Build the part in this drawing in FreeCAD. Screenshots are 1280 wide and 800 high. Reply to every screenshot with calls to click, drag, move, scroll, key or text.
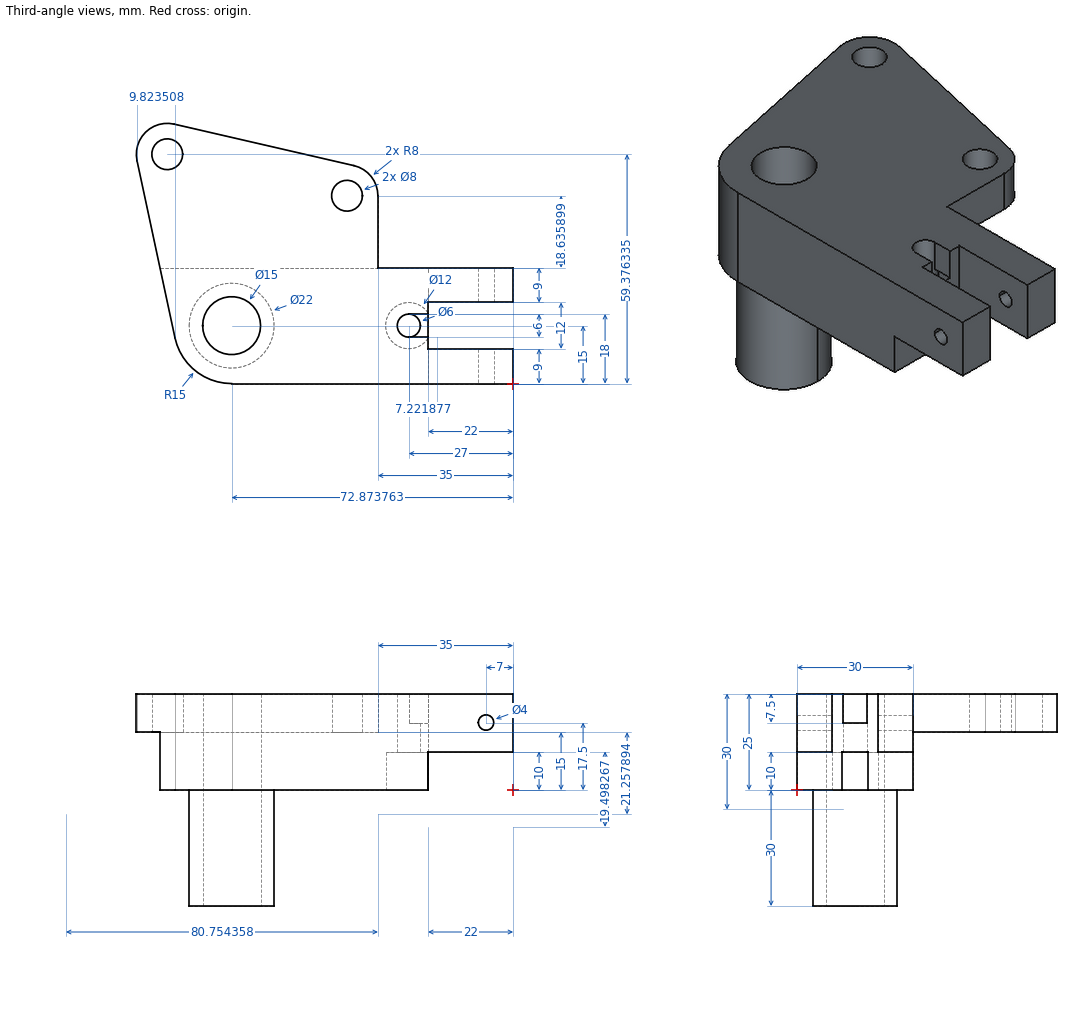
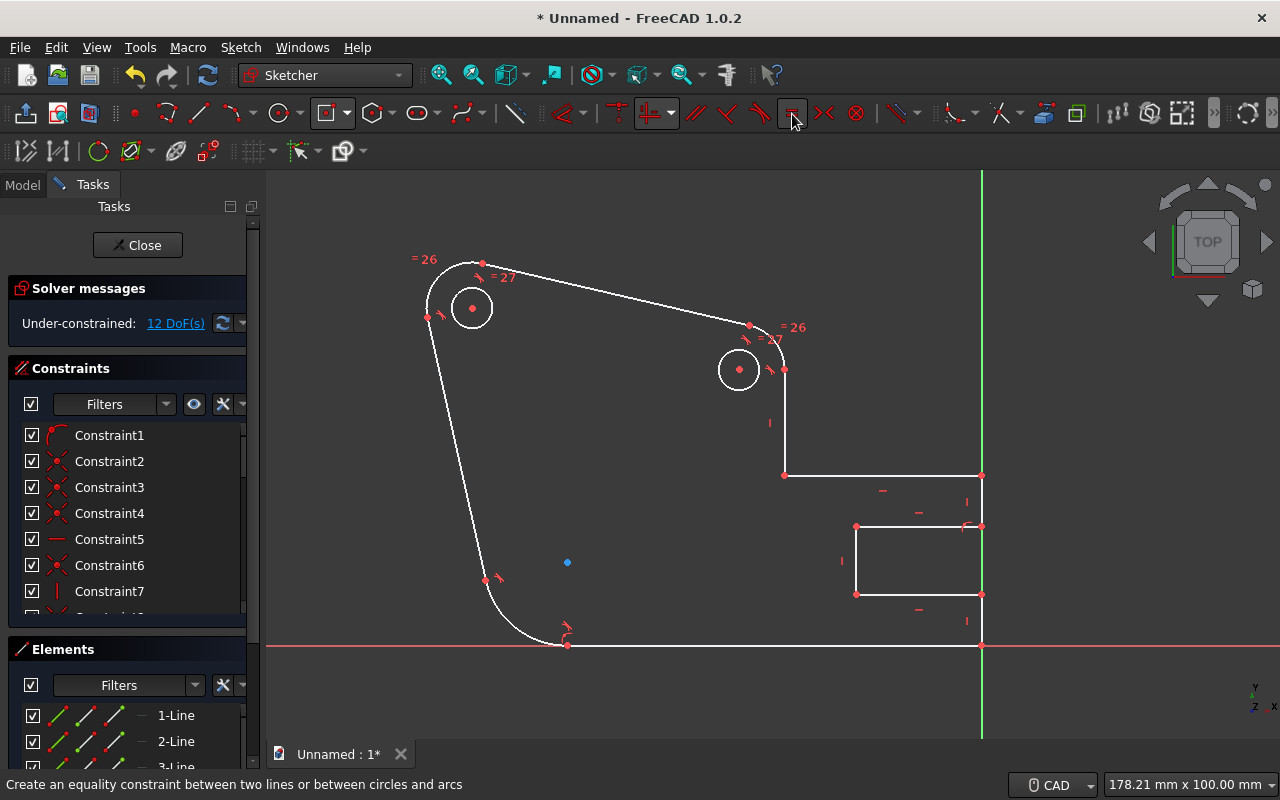
click(562, 114)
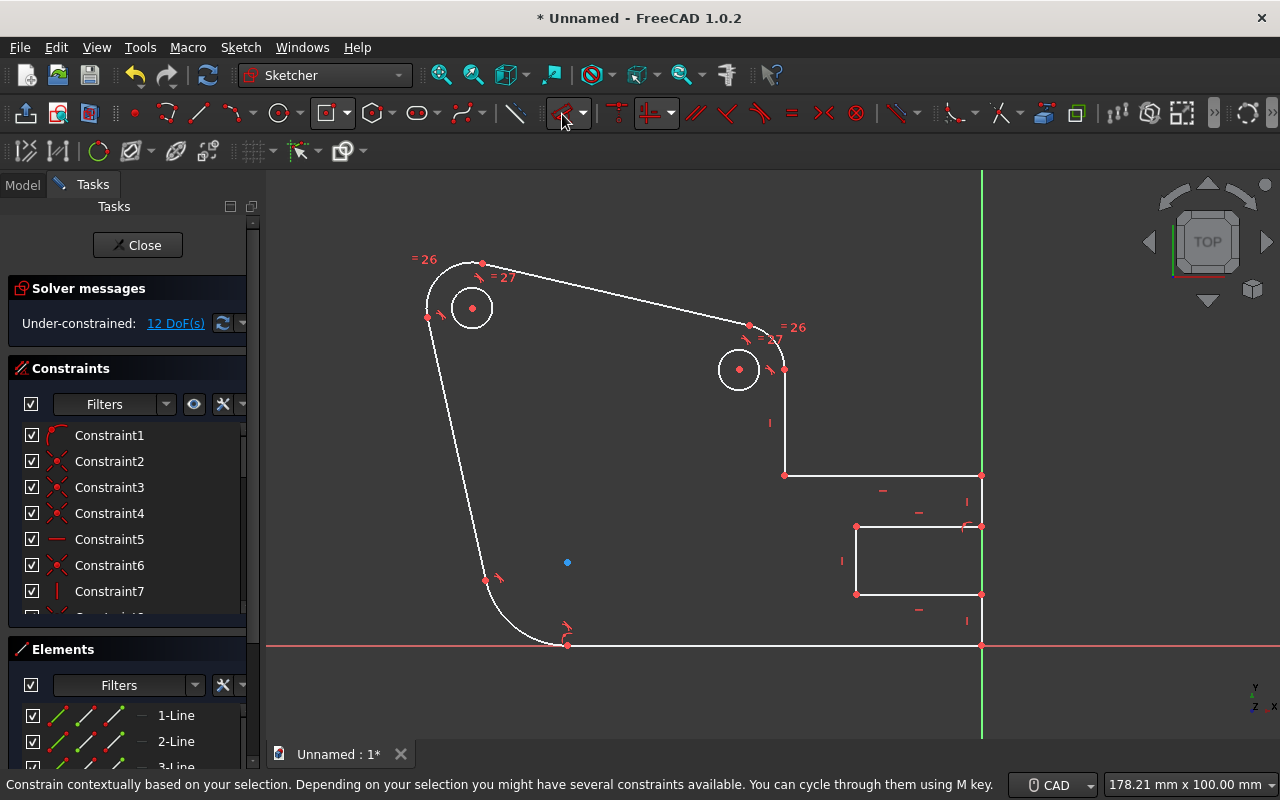
click(781, 352)
click(810, 339)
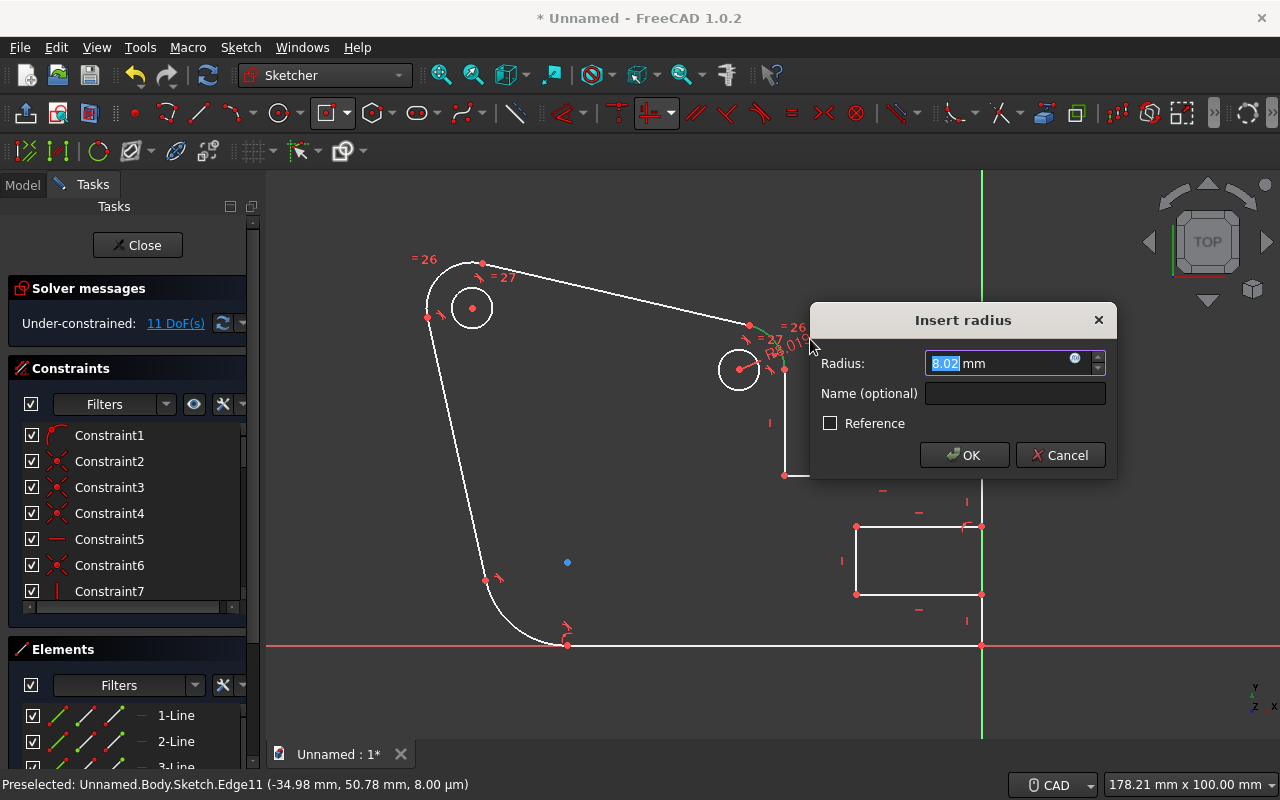
text(8)
key(Return)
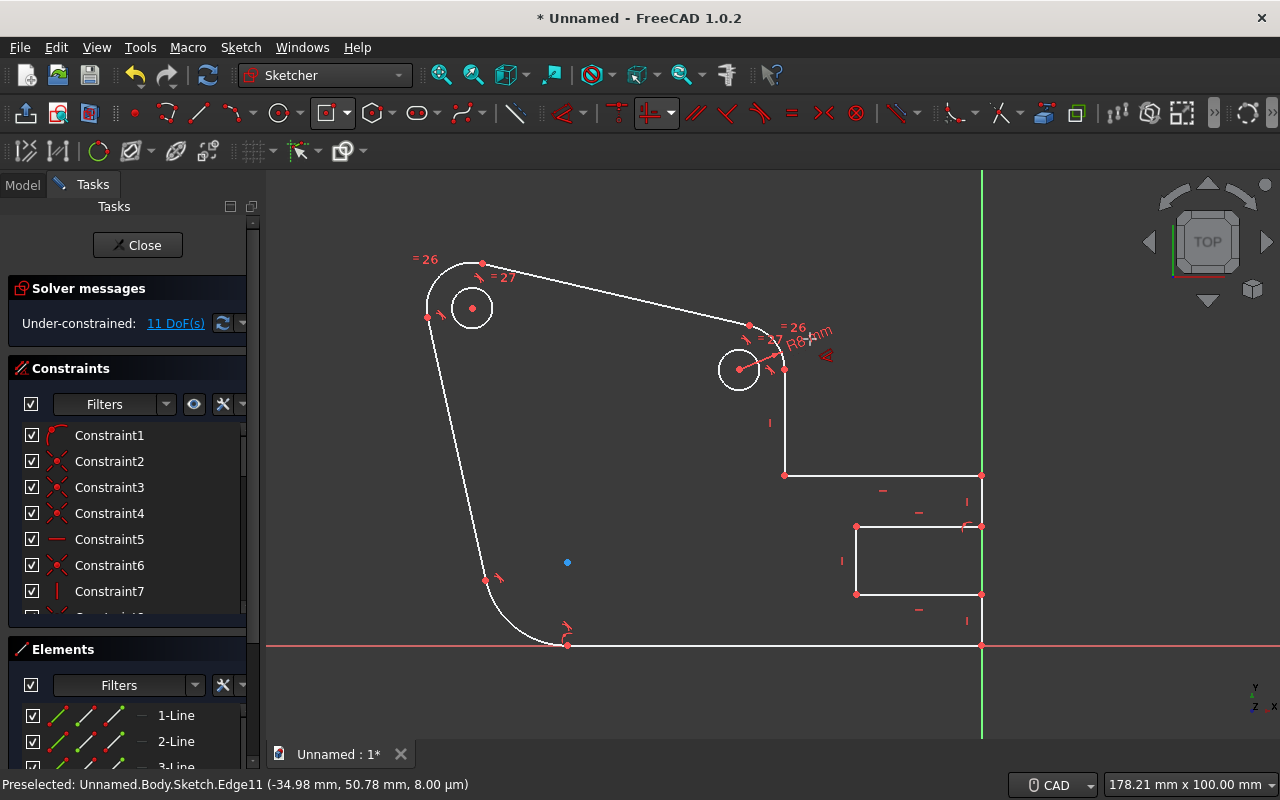
click(500, 611)
click(474, 630)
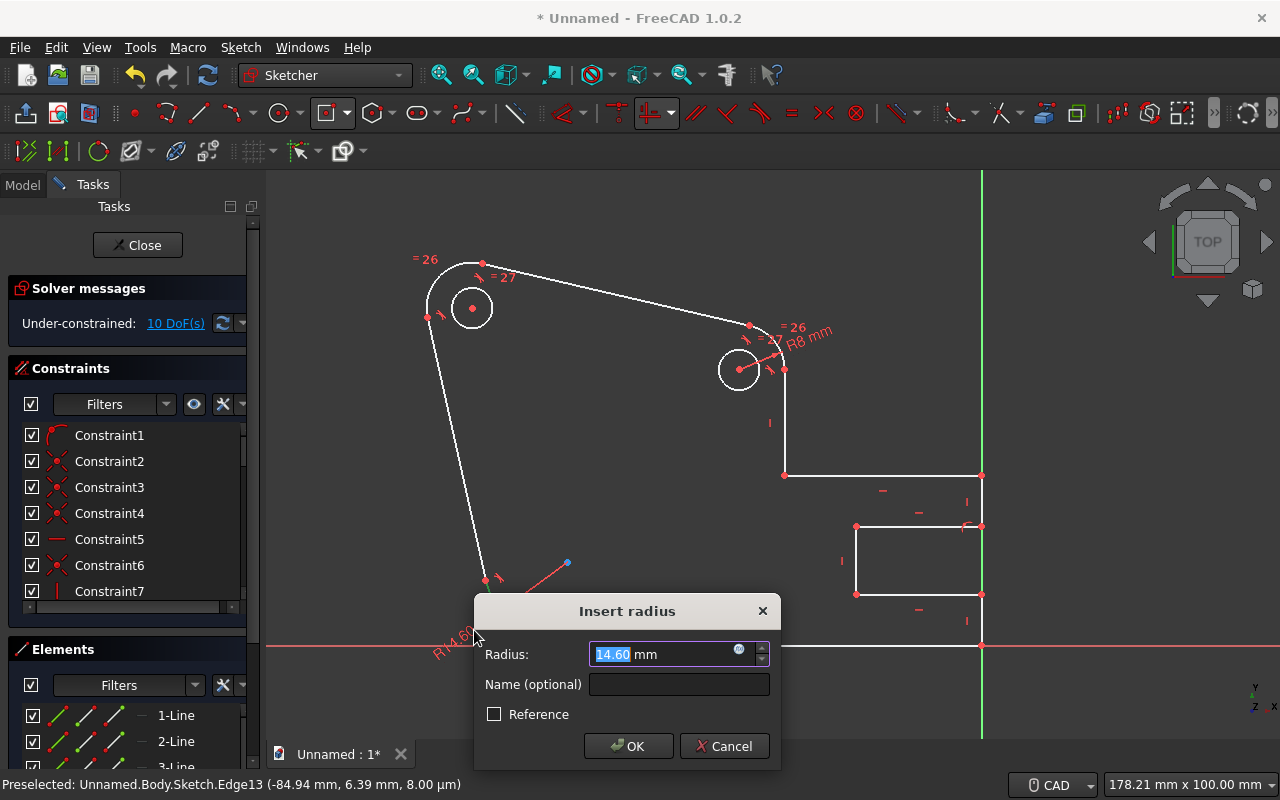
text(15)
key(Return)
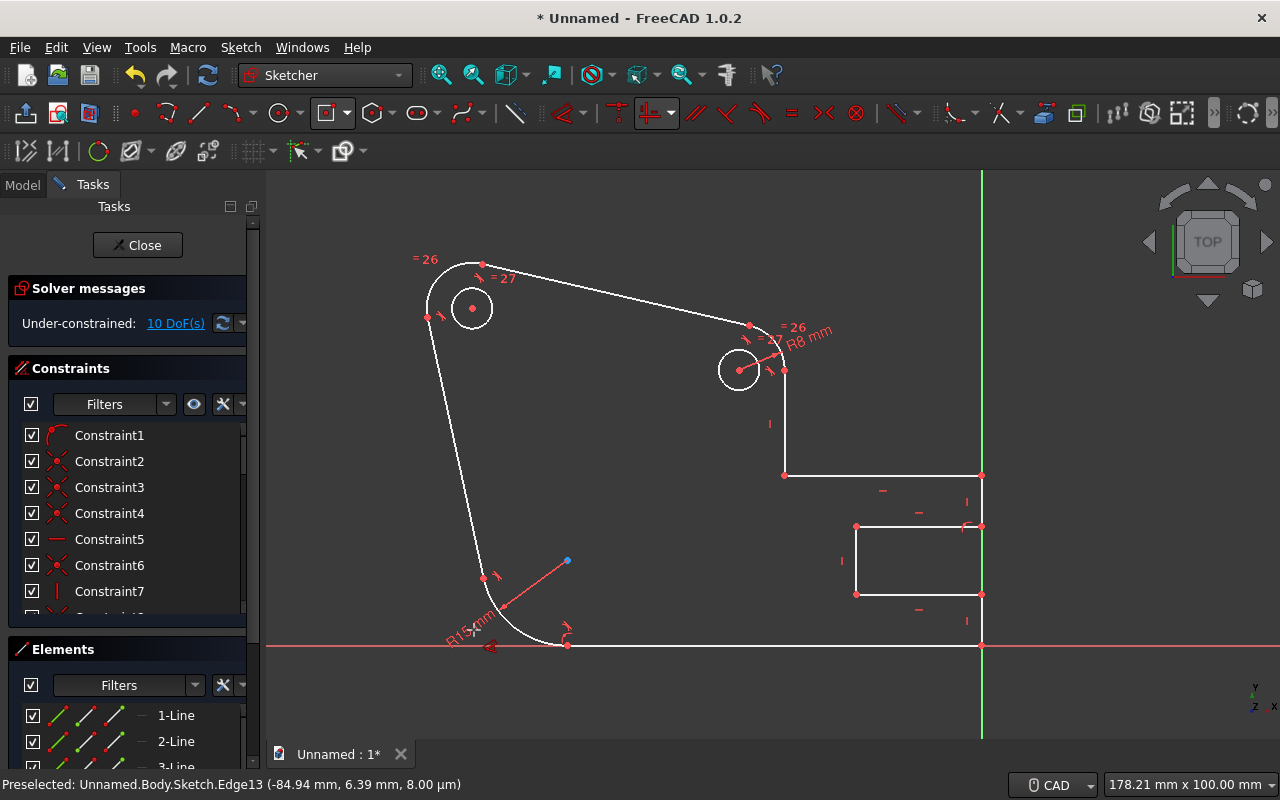
click(753, 356)
click(702, 334)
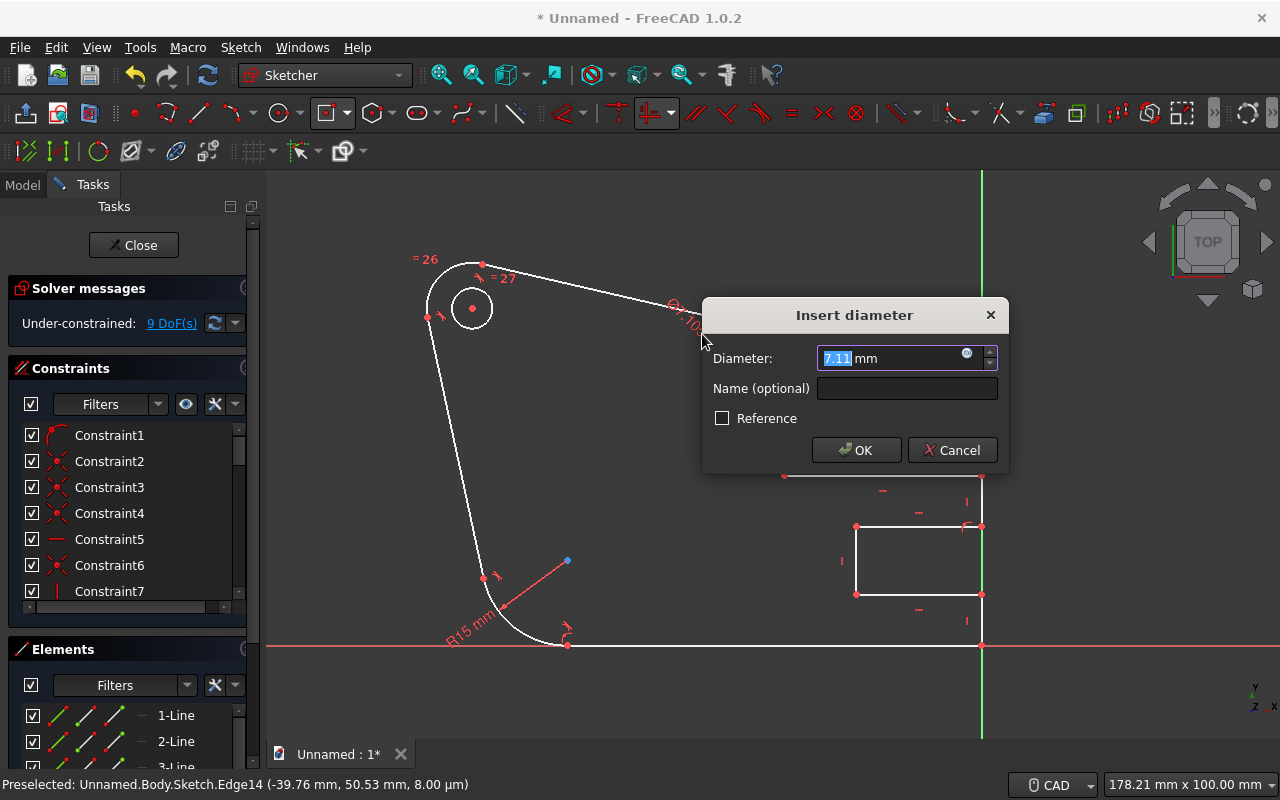
text(8)
key(Return)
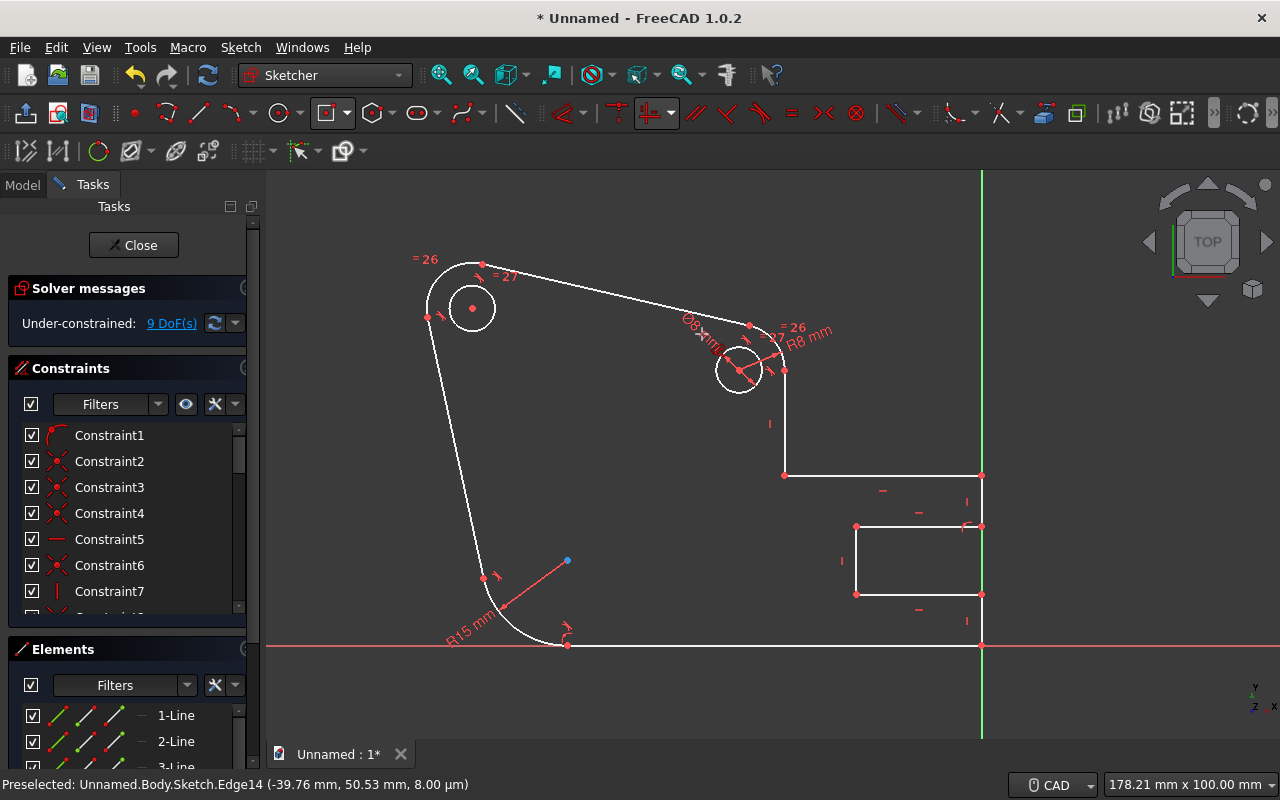
click(982, 630)
click(1016, 620)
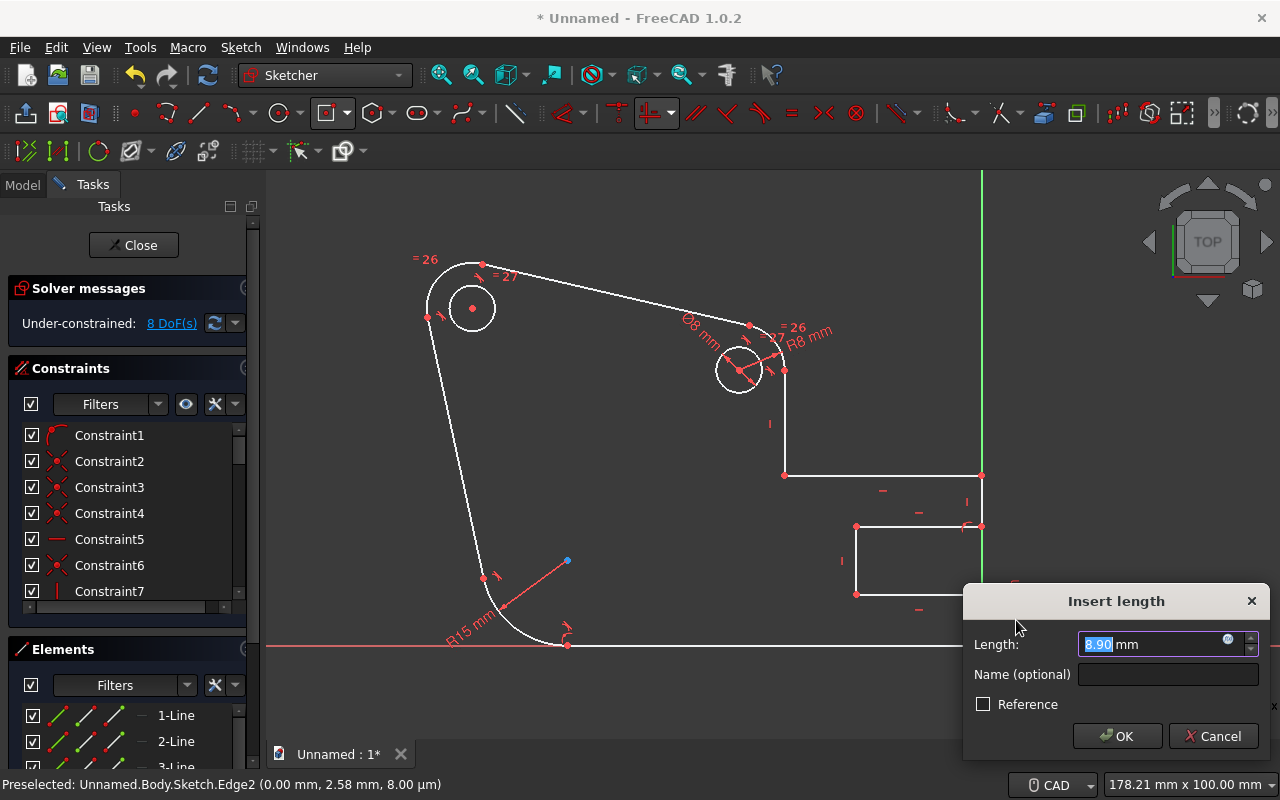
text(9)
key(Return)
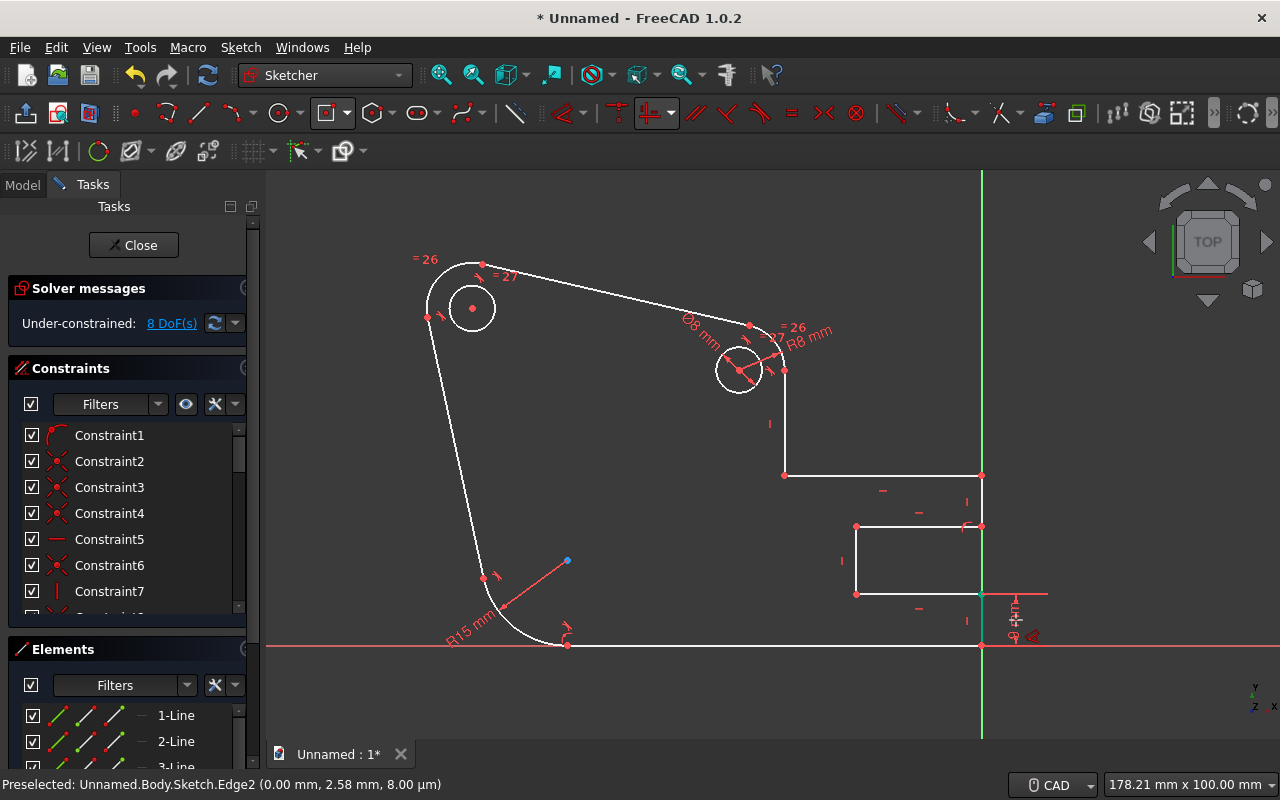
click(982, 512)
click(1016, 501)